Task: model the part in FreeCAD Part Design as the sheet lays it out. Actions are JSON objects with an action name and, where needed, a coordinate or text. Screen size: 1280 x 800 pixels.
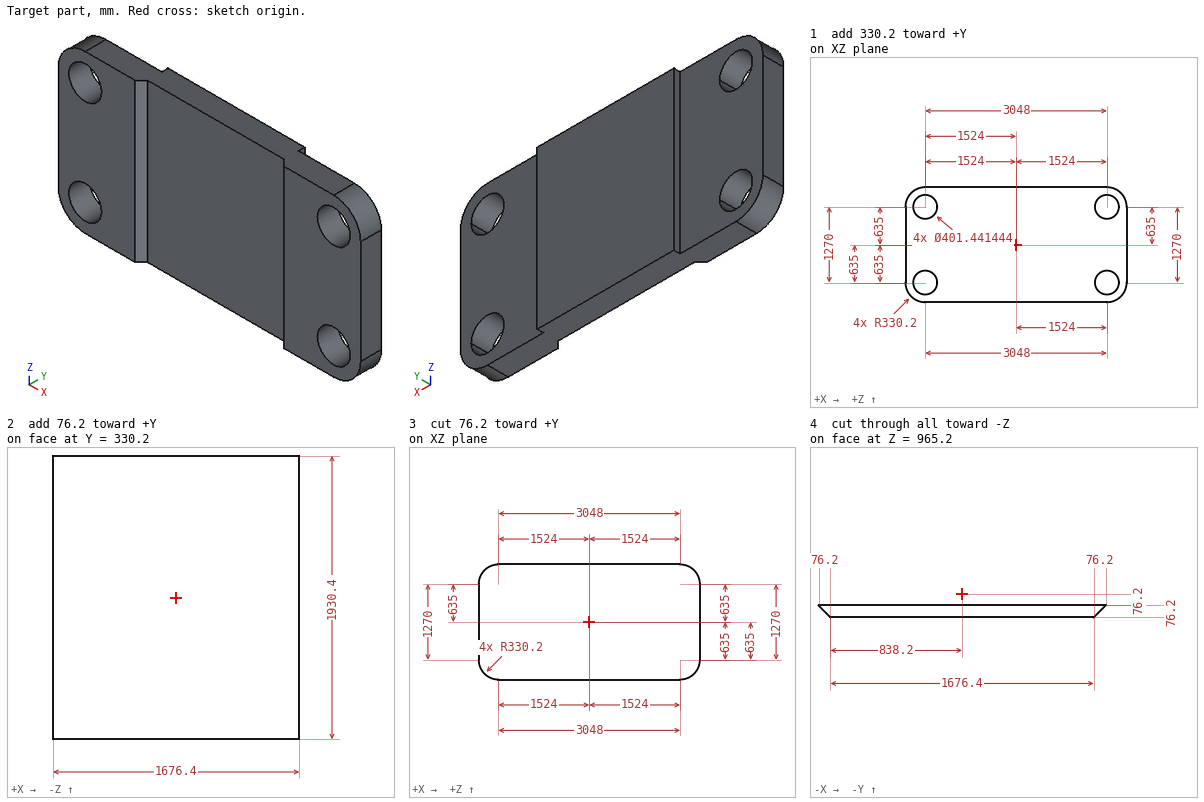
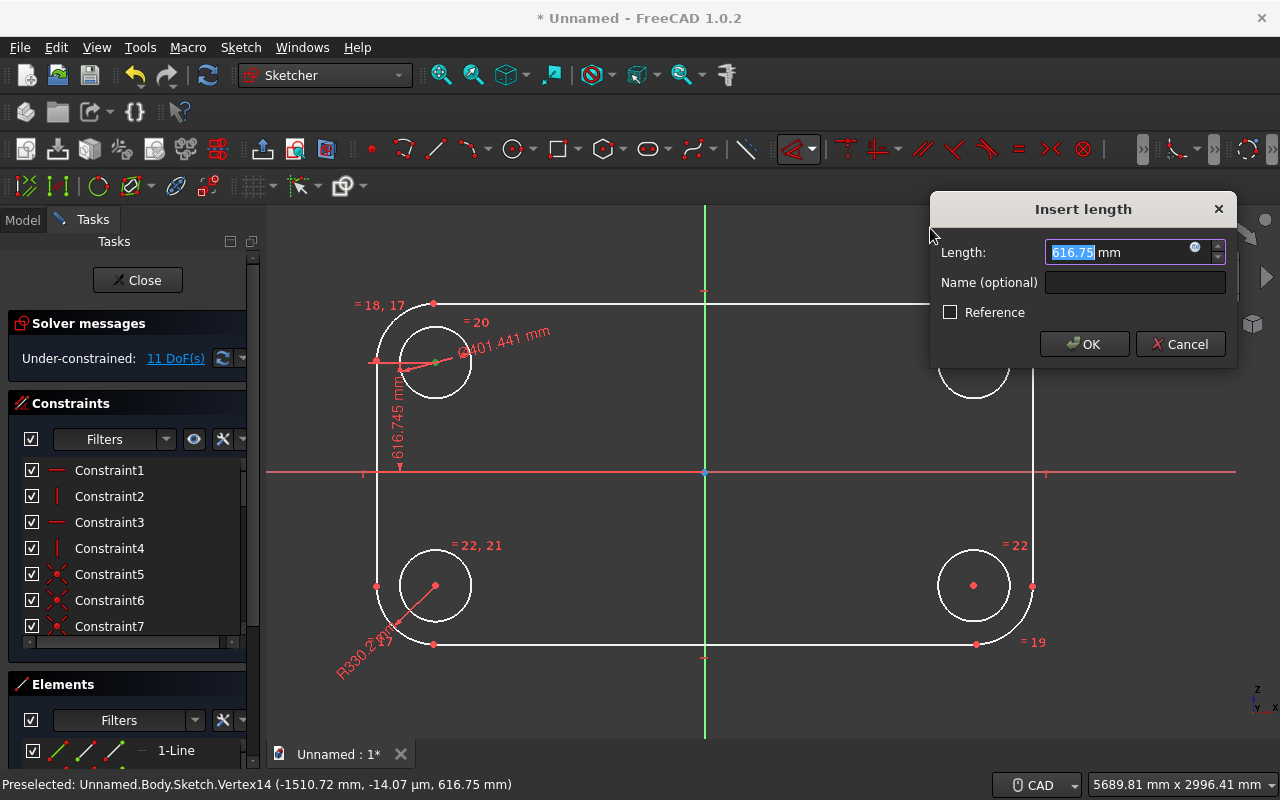
{"action": "type", "text": "635"}
{"action": "key", "text": "Return"}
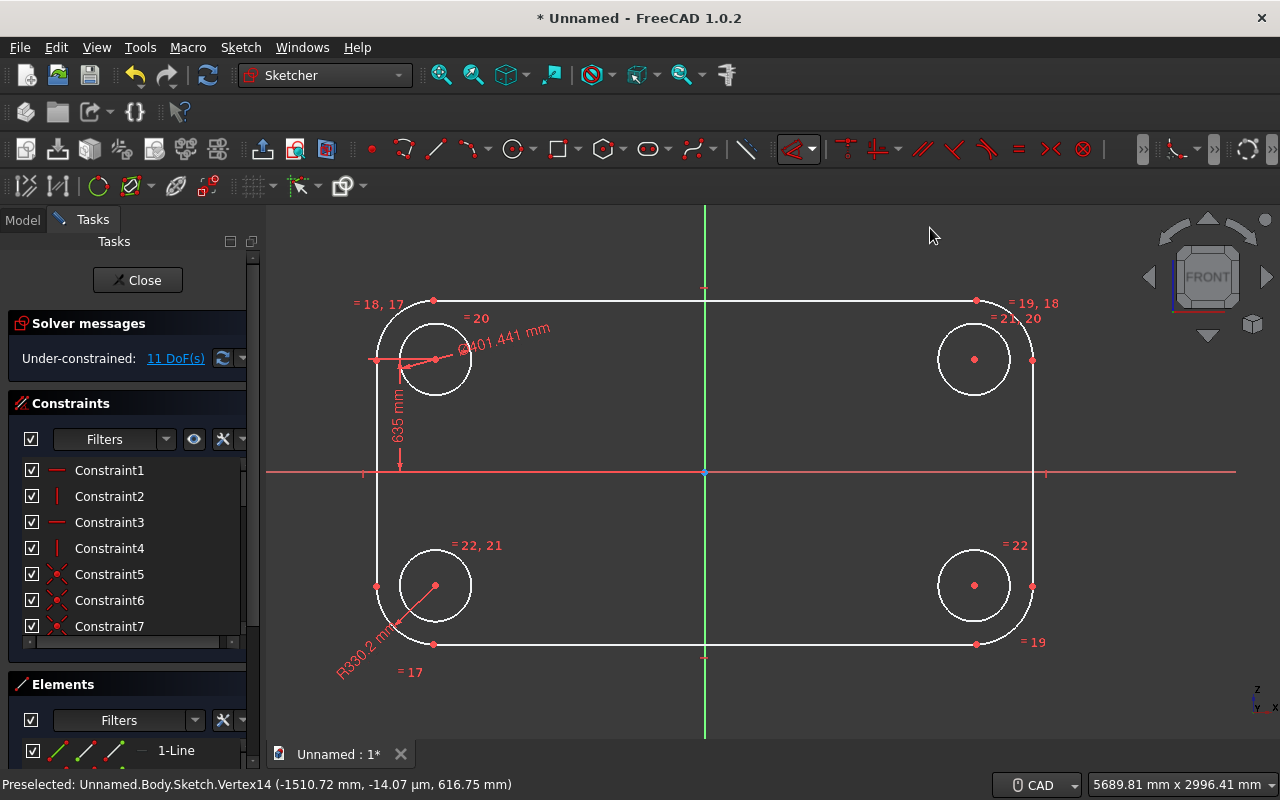
{"action": "left_click", "coordinate": [436, 586]}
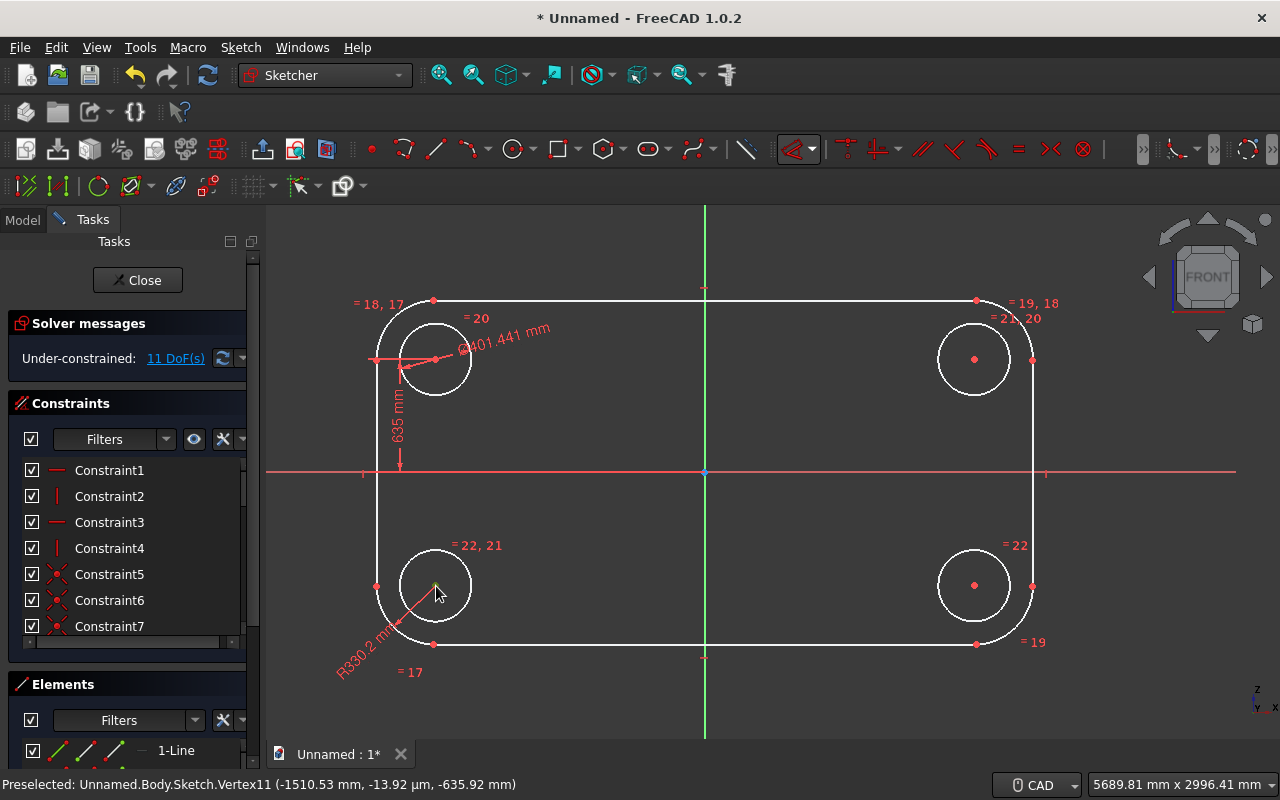
{"action": "key", "text": "i"}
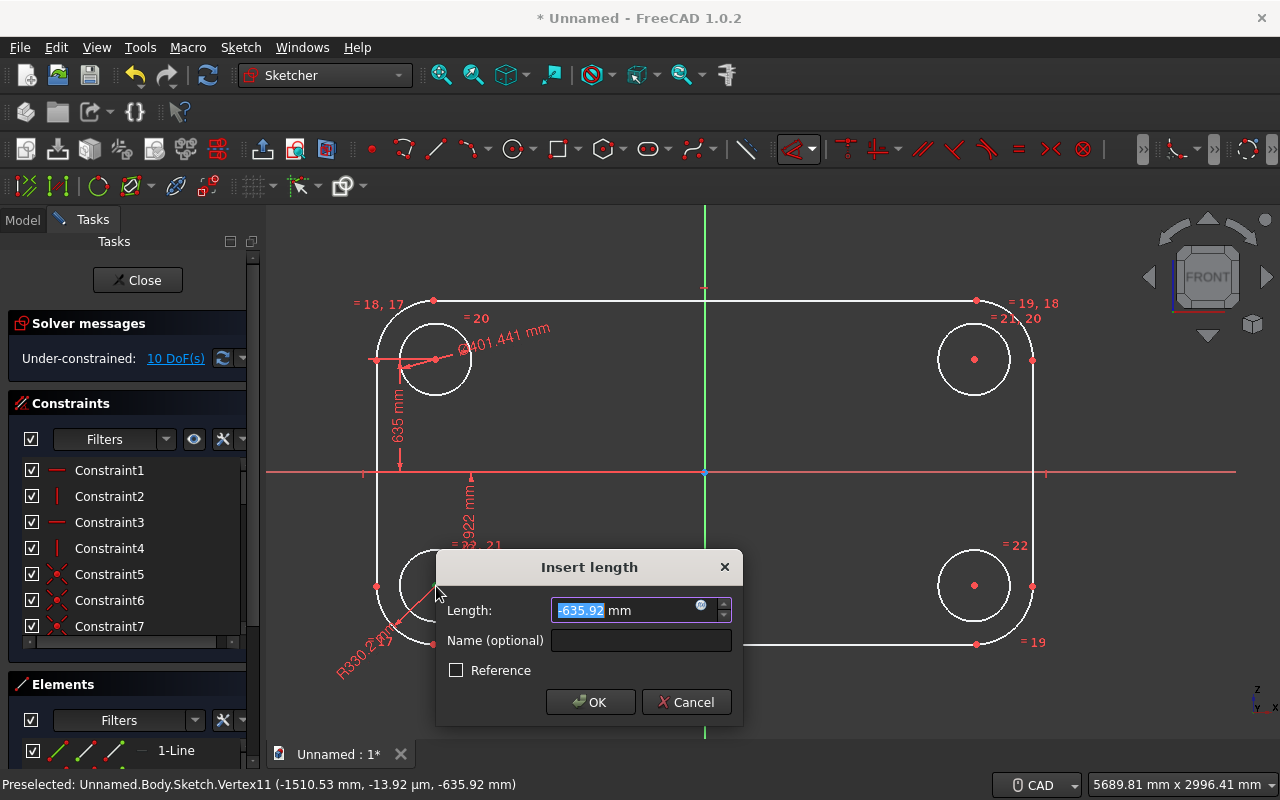
{"action": "type", "text": "-635"}
{"action": "key", "text": "Return"}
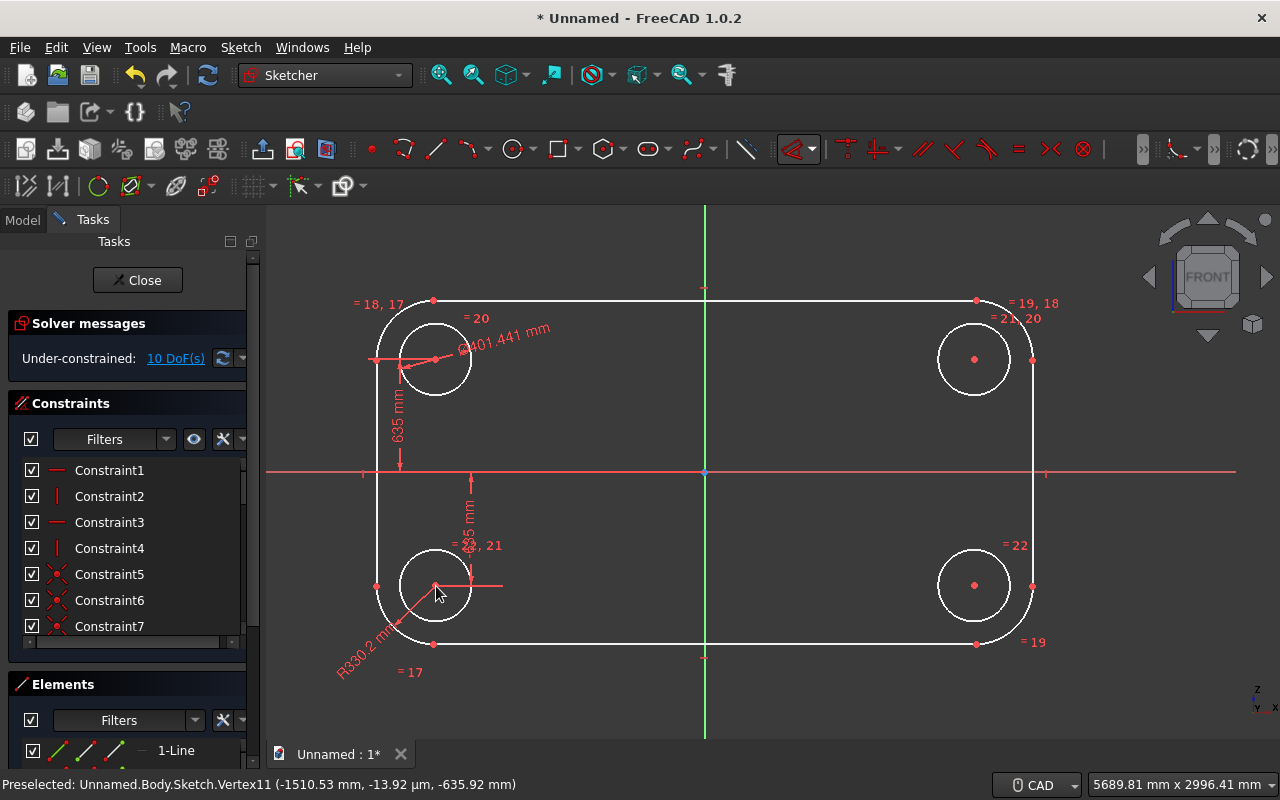
{"action": "left_click", "coordinate": [813, 644]}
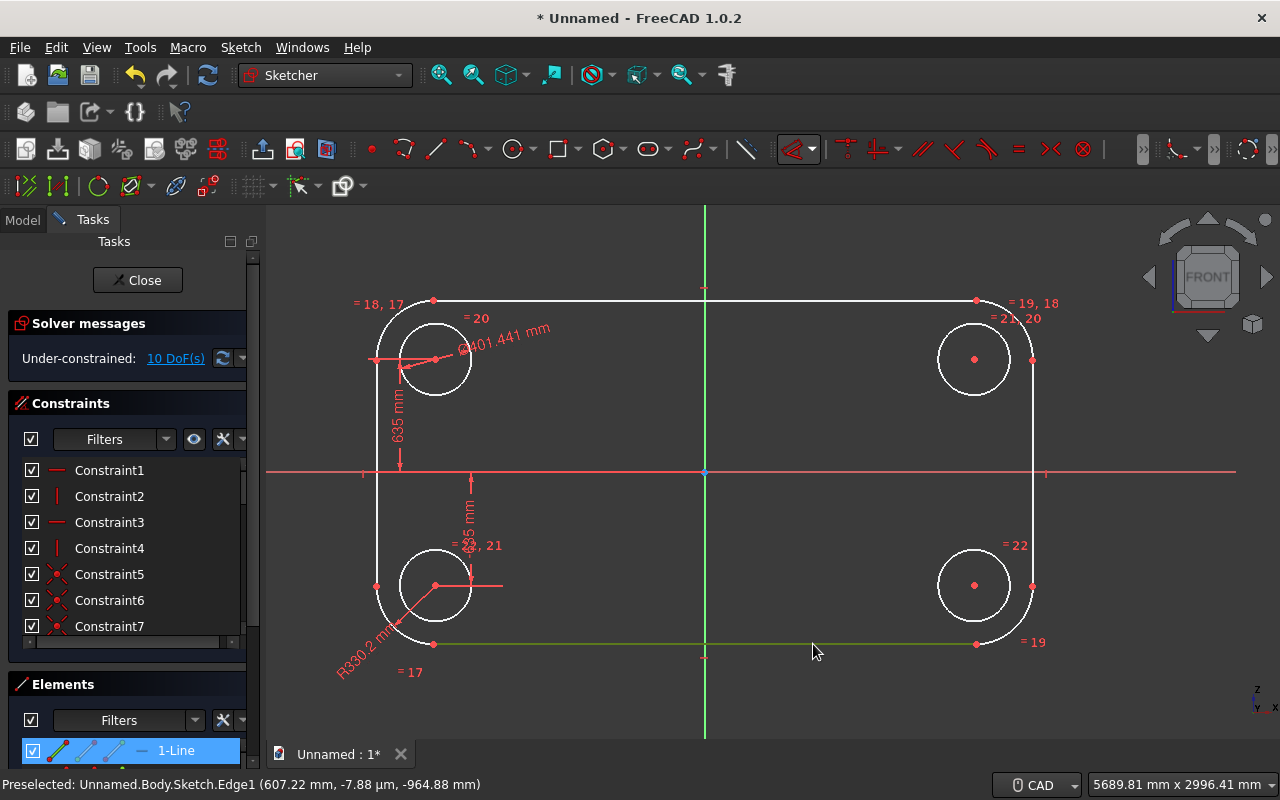
{"action": "left_click", "coordinate": [814, 150]}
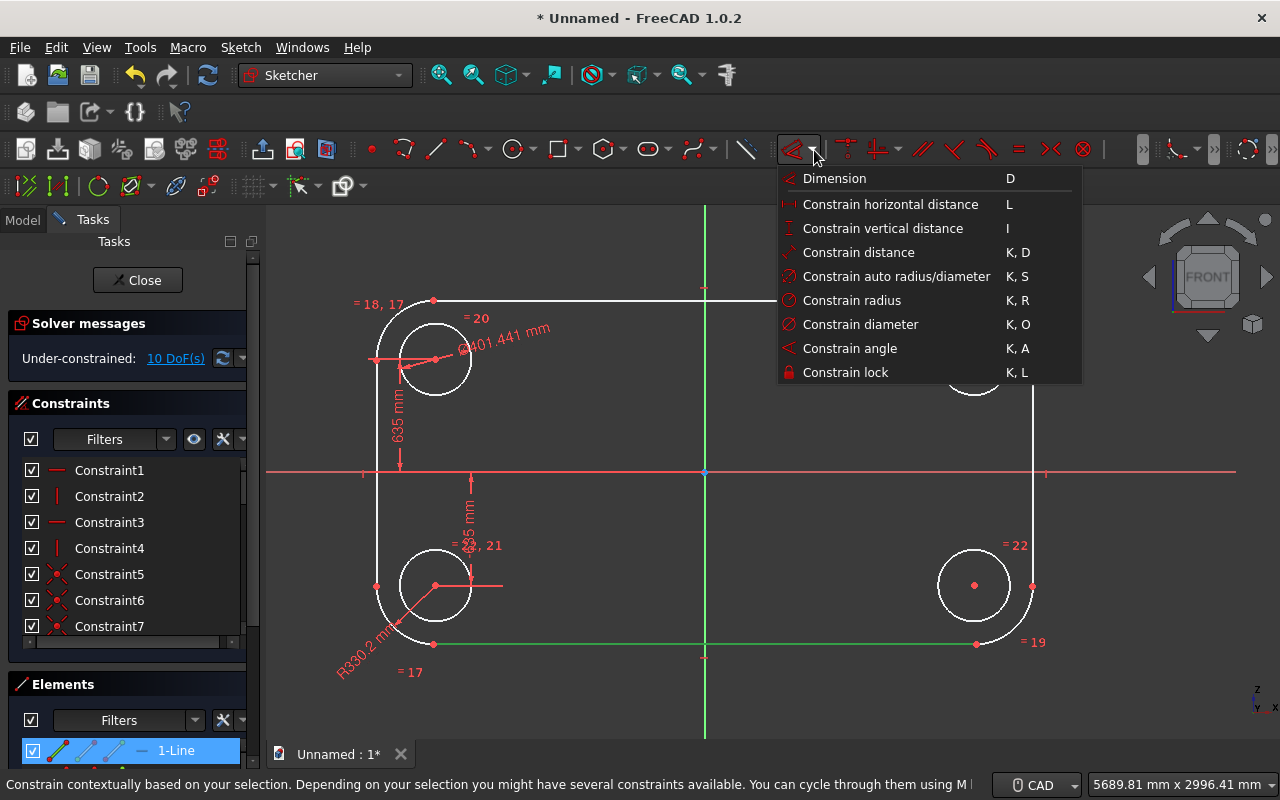
{"action": "left_click", "coordinate": [930, 204]}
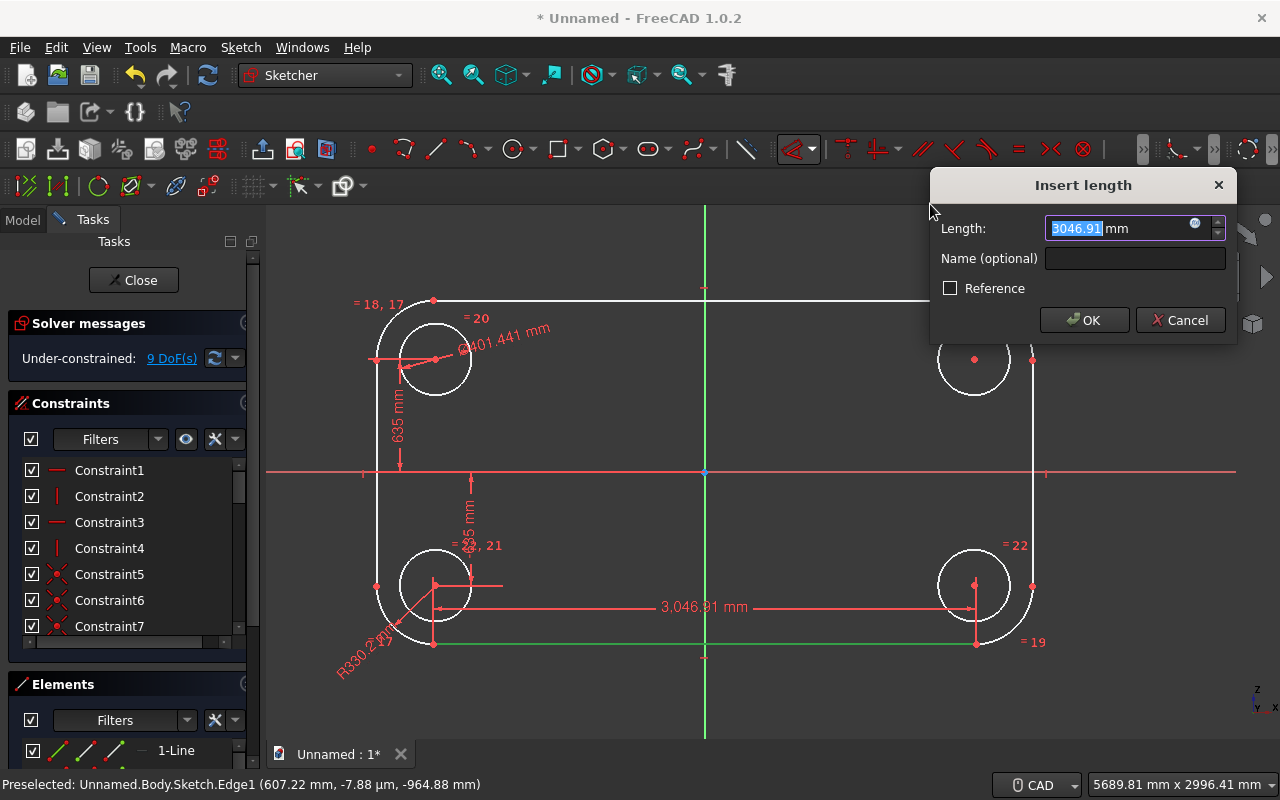
{"action": "type", "text": "3048"}
{"action": "key", "text": "Return"}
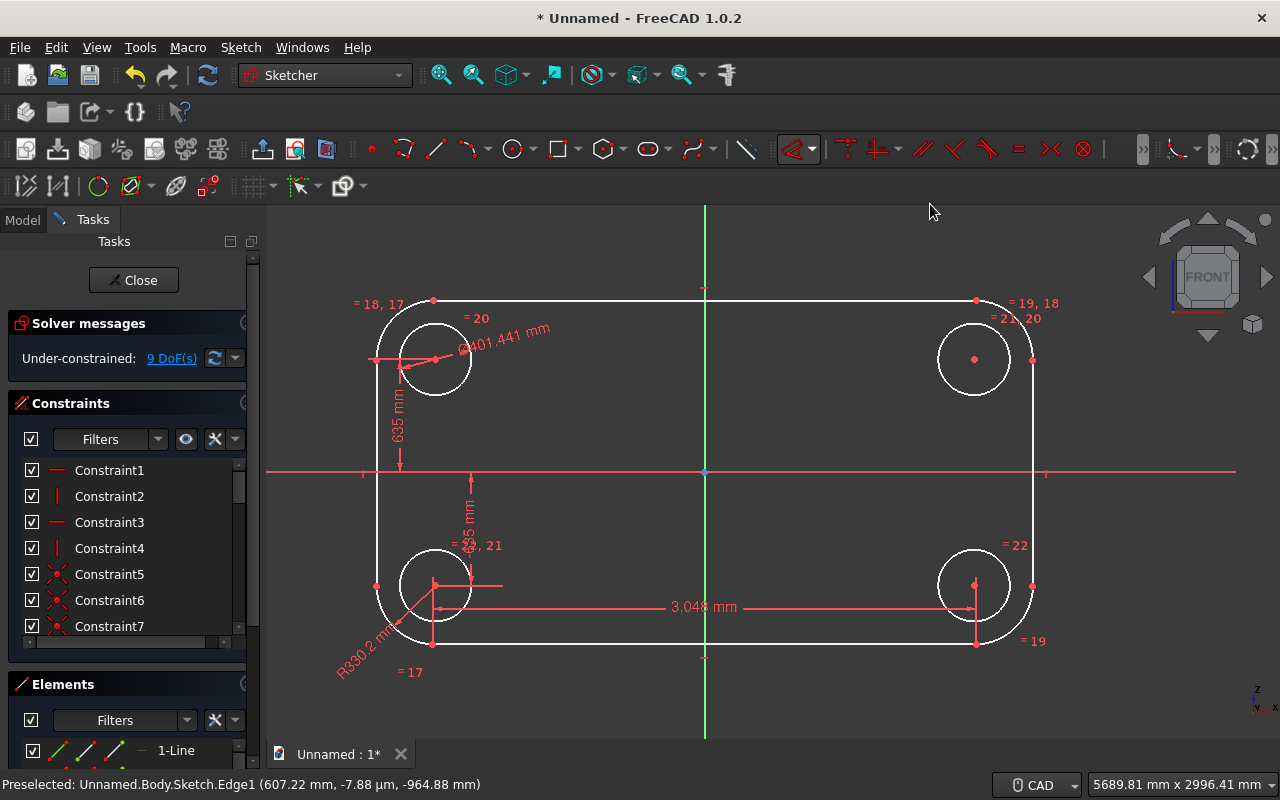
{"action": "left_click", "coordinate": [377, 519]}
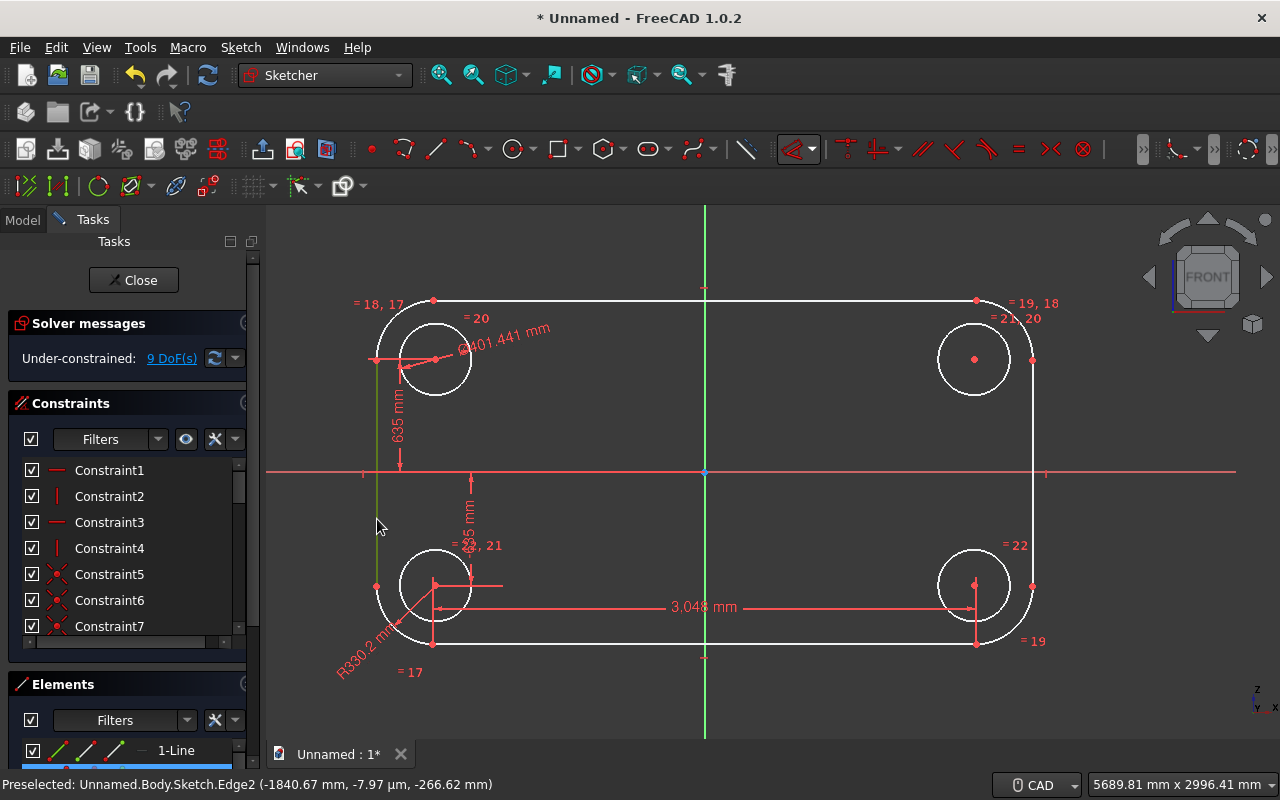
{"action": "key", "text": "i"}